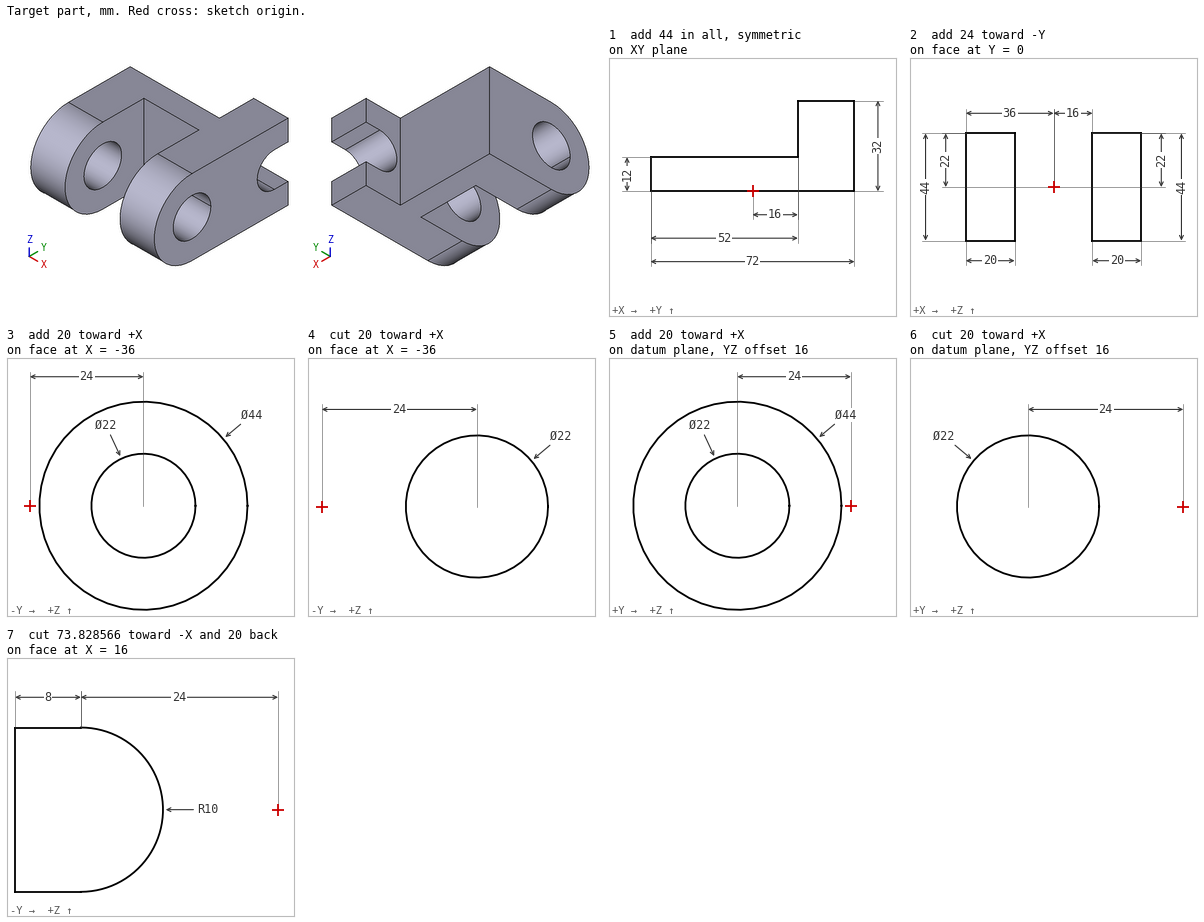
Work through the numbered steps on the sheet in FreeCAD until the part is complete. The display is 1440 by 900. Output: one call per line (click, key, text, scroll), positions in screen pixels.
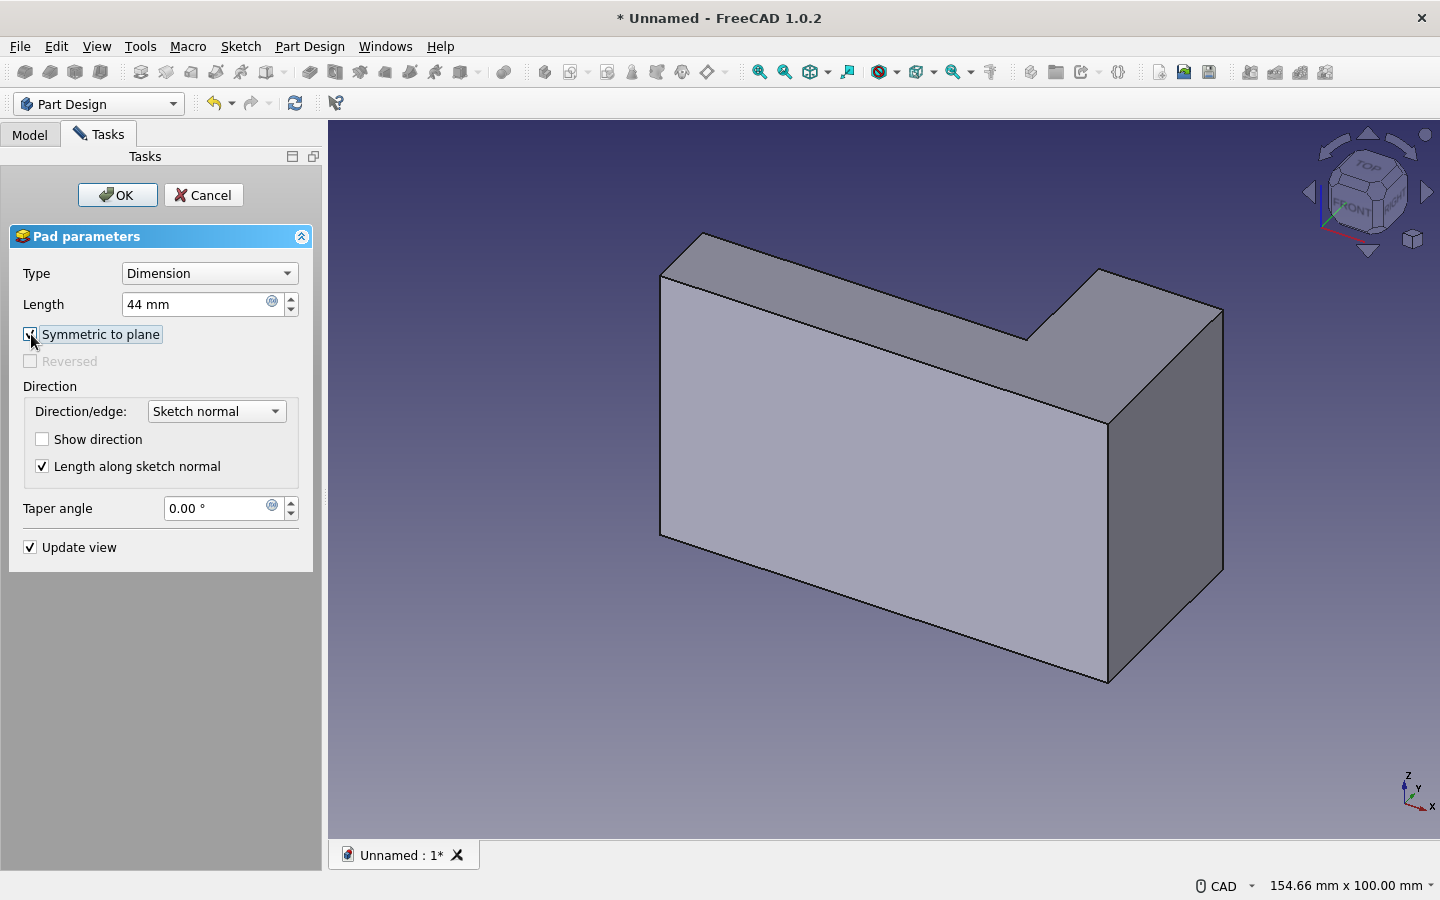
click(118, 195)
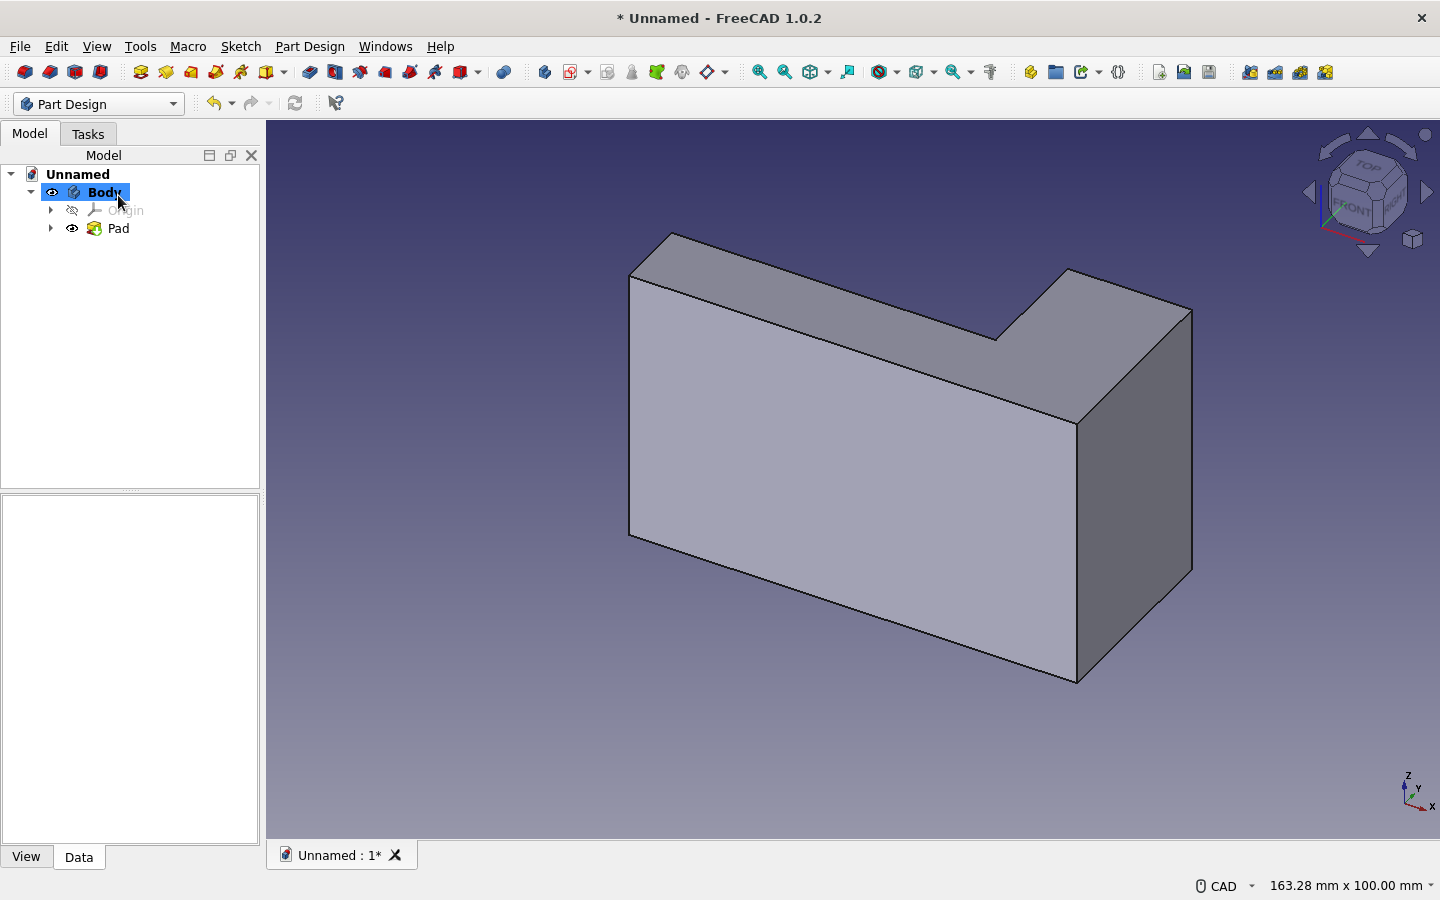
click(917, 500)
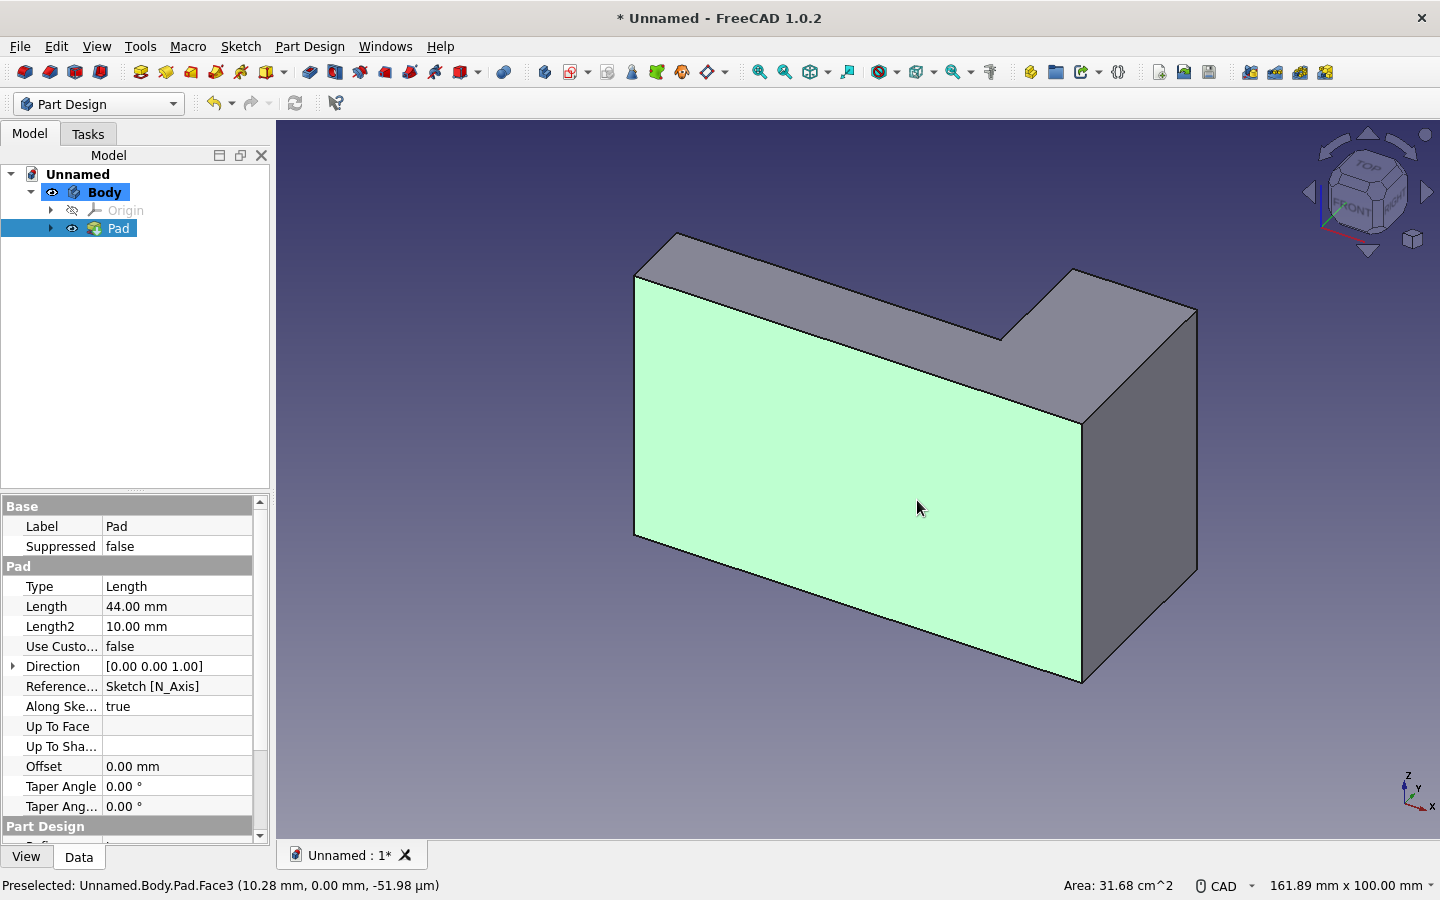
click(570, 72)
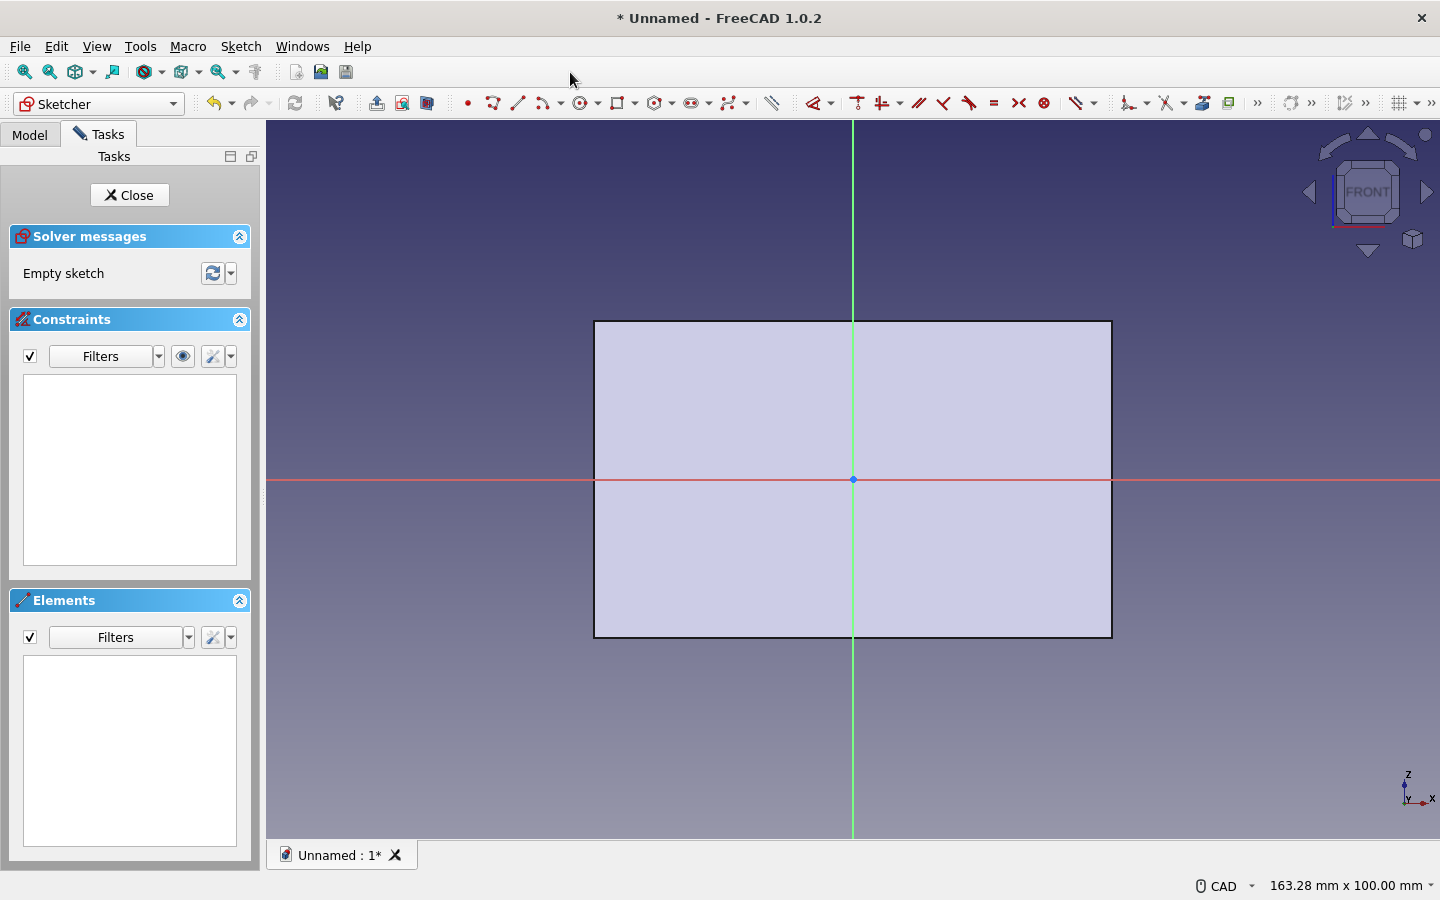
click(616, 104)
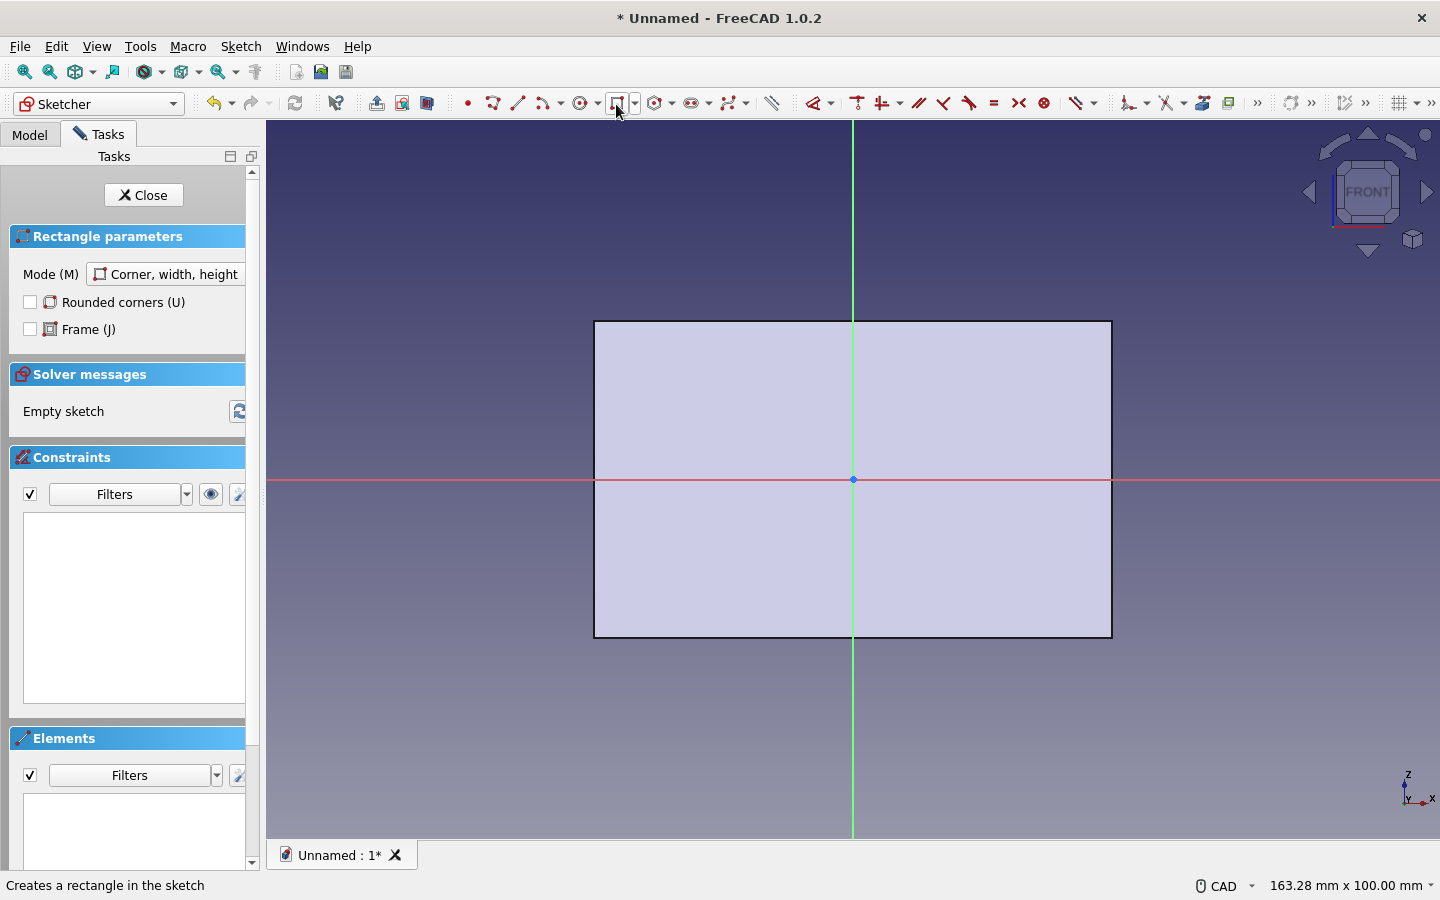
click(594, 321)
click(738, 638)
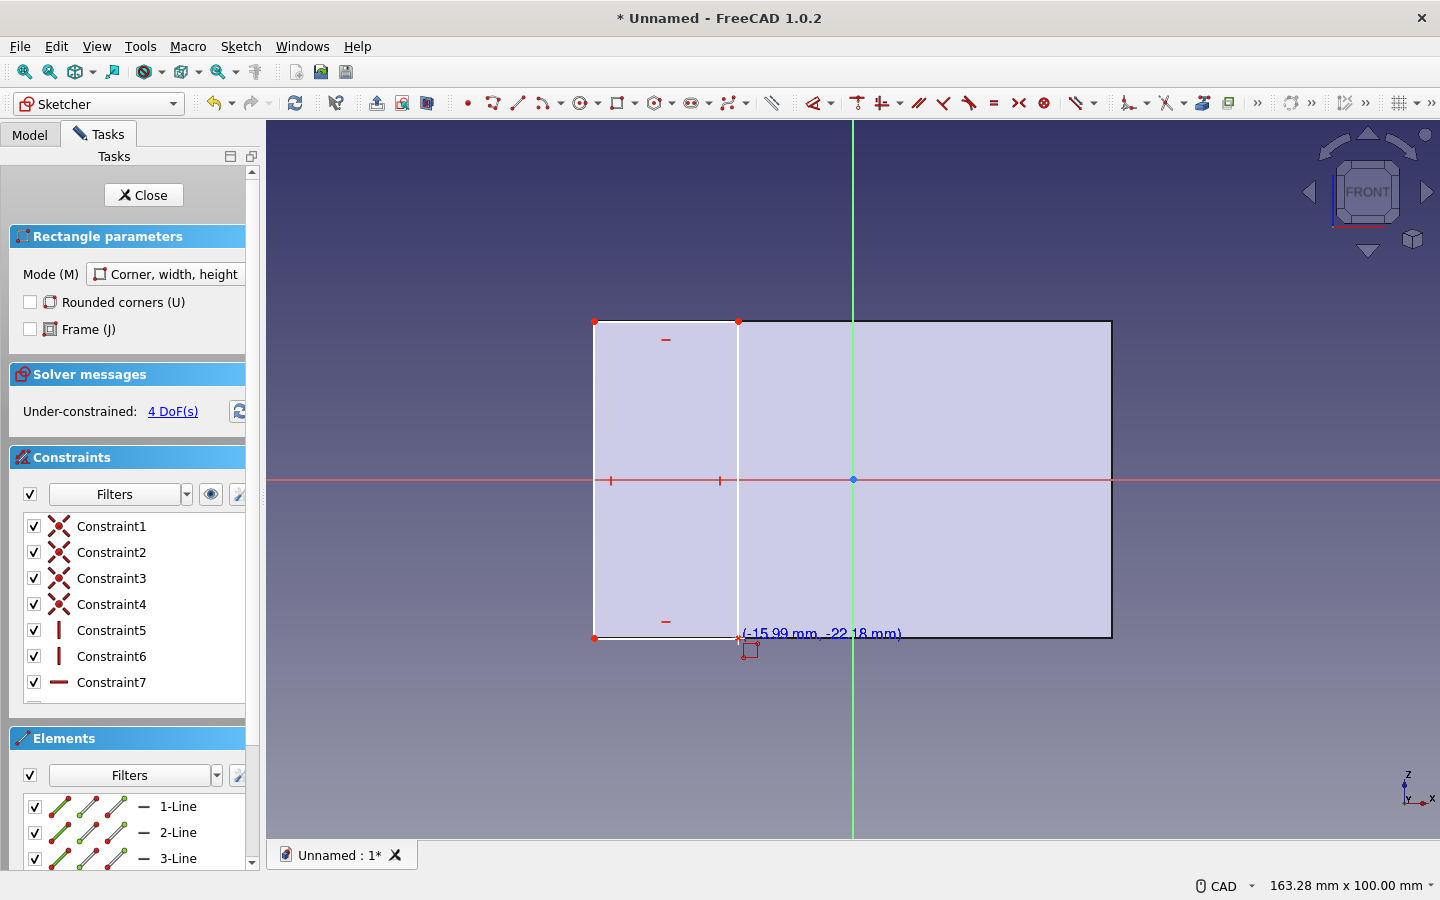
click(968, 321)
click(1112, 638)
key(Escape)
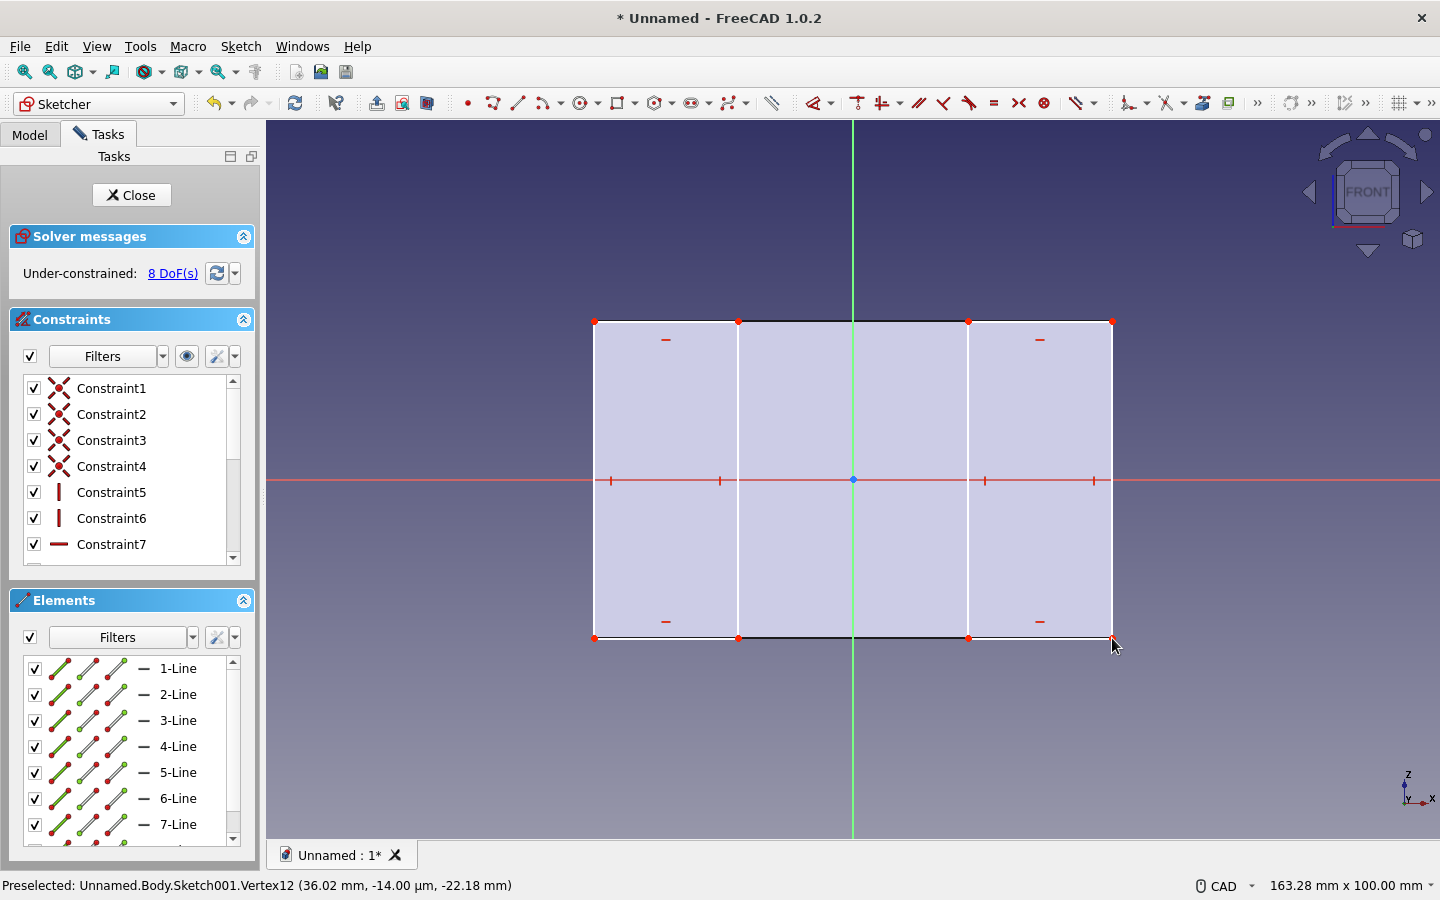
click(812, 104)